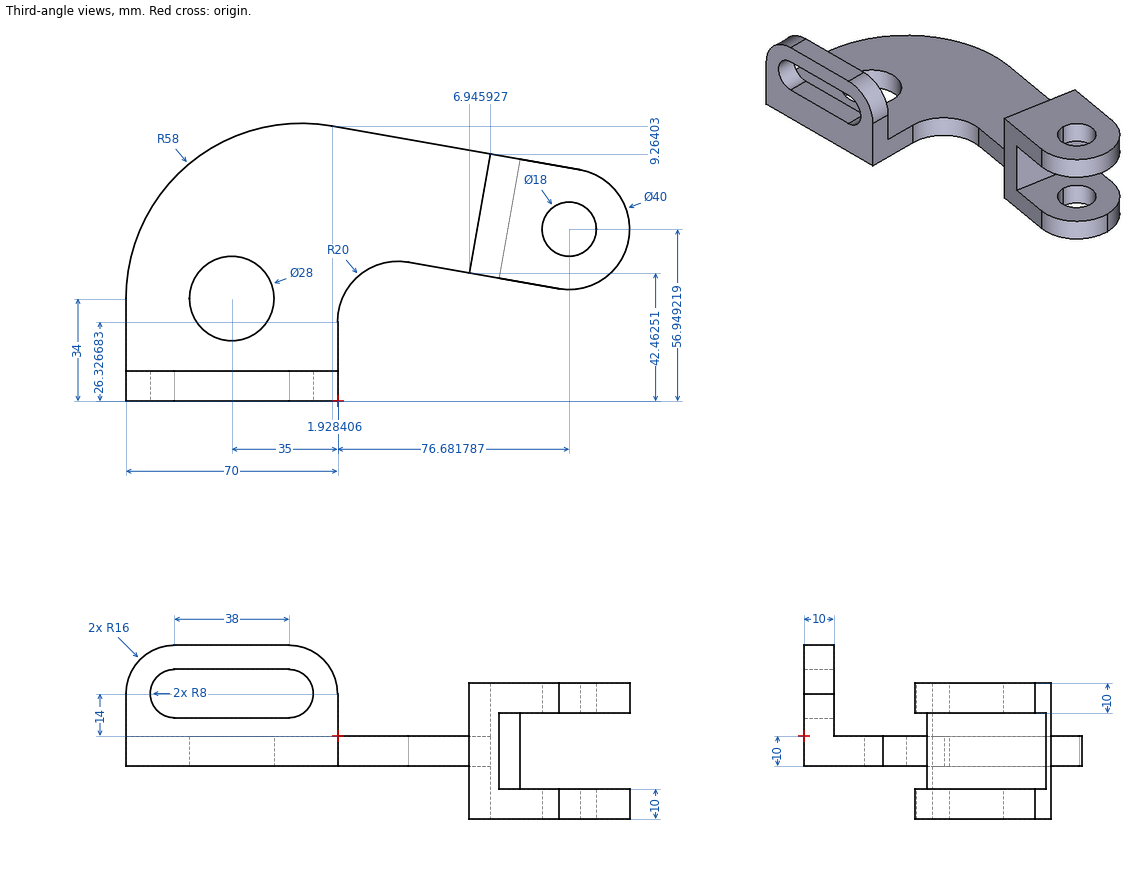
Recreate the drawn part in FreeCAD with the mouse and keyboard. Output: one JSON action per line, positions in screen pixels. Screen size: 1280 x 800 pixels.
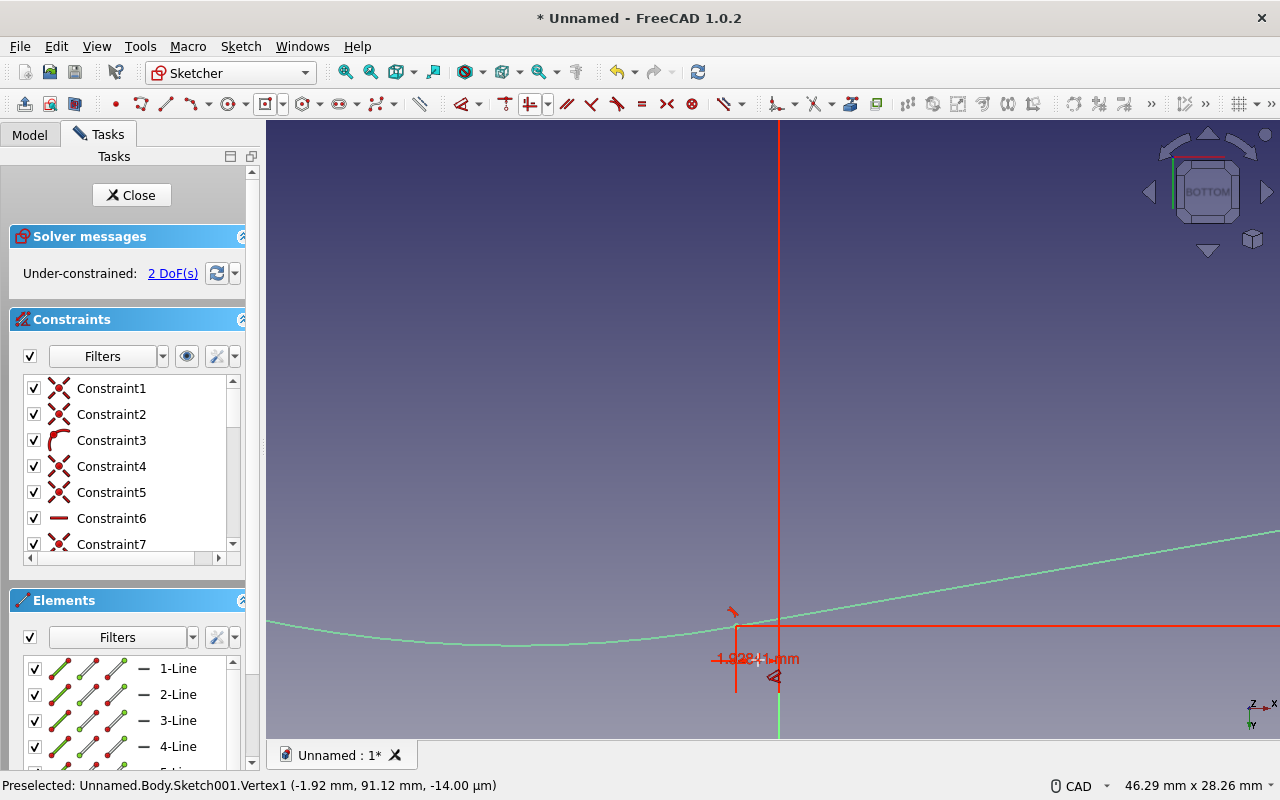
{"action": "scroll", "coordinate": [739, 632], "scroll_direction": "down", "scroll_amount": 8}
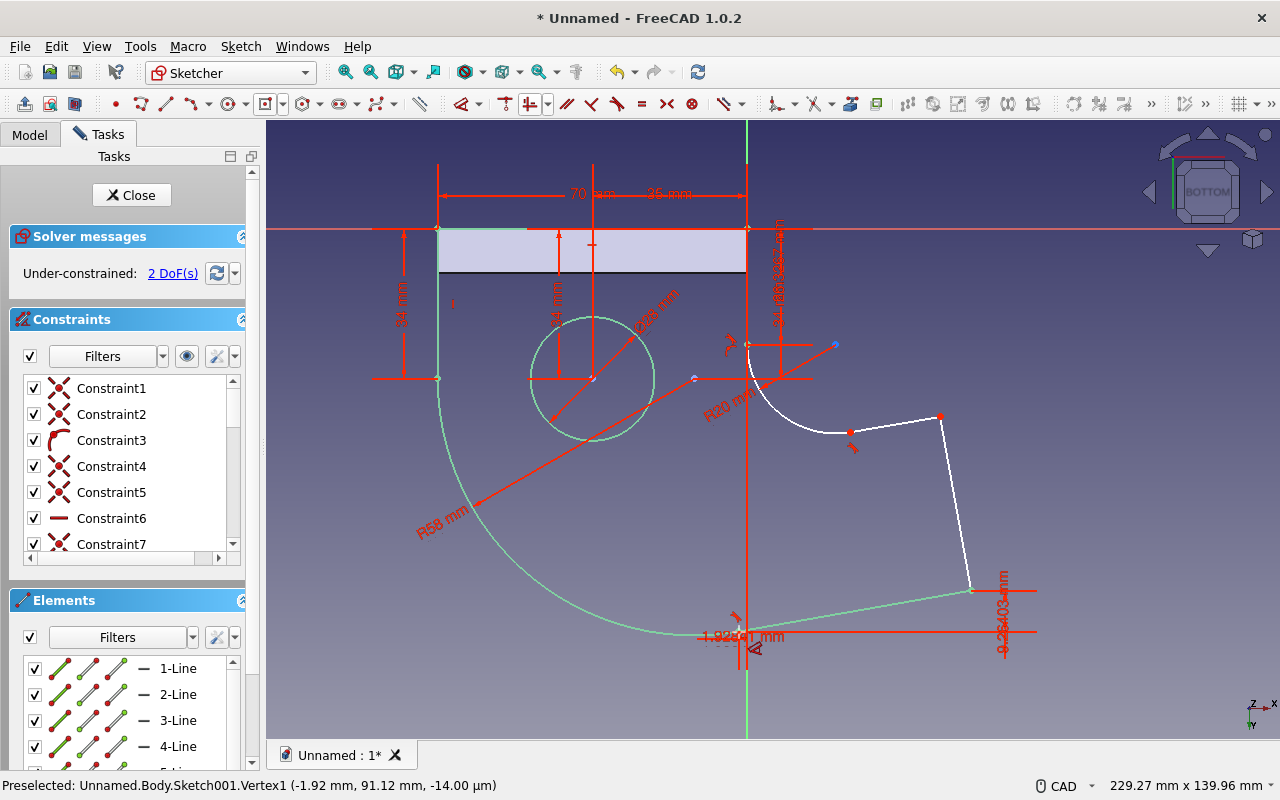
{"action": "left_click", "coordinate": [940, 417]}
{"action": "left_click", "coordinate": [974, 323]}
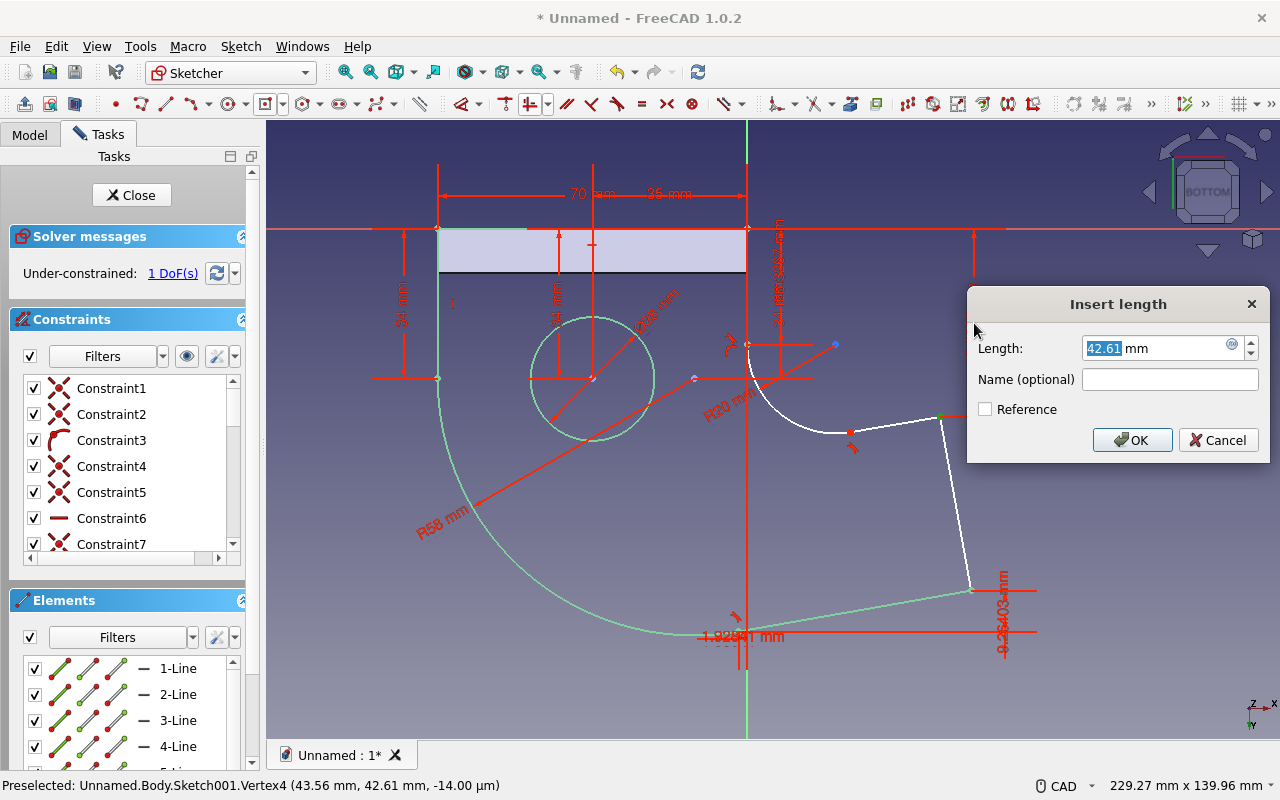
{"action": "type", "text": "42.46251"}
{"action": "key", "text": "Return"}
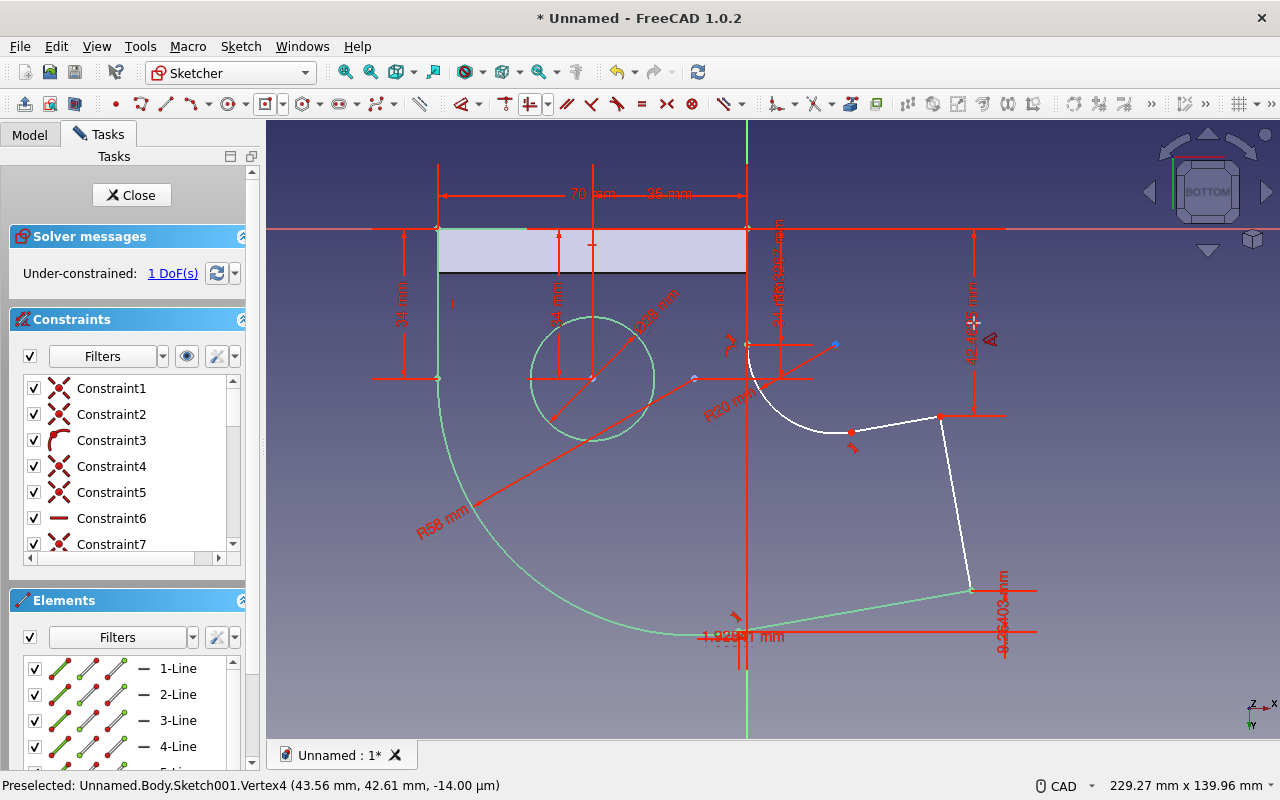
{"action": "scroll", "coordinate": [962, 538], "scroll_direction": "up", "scroll_amount": 2}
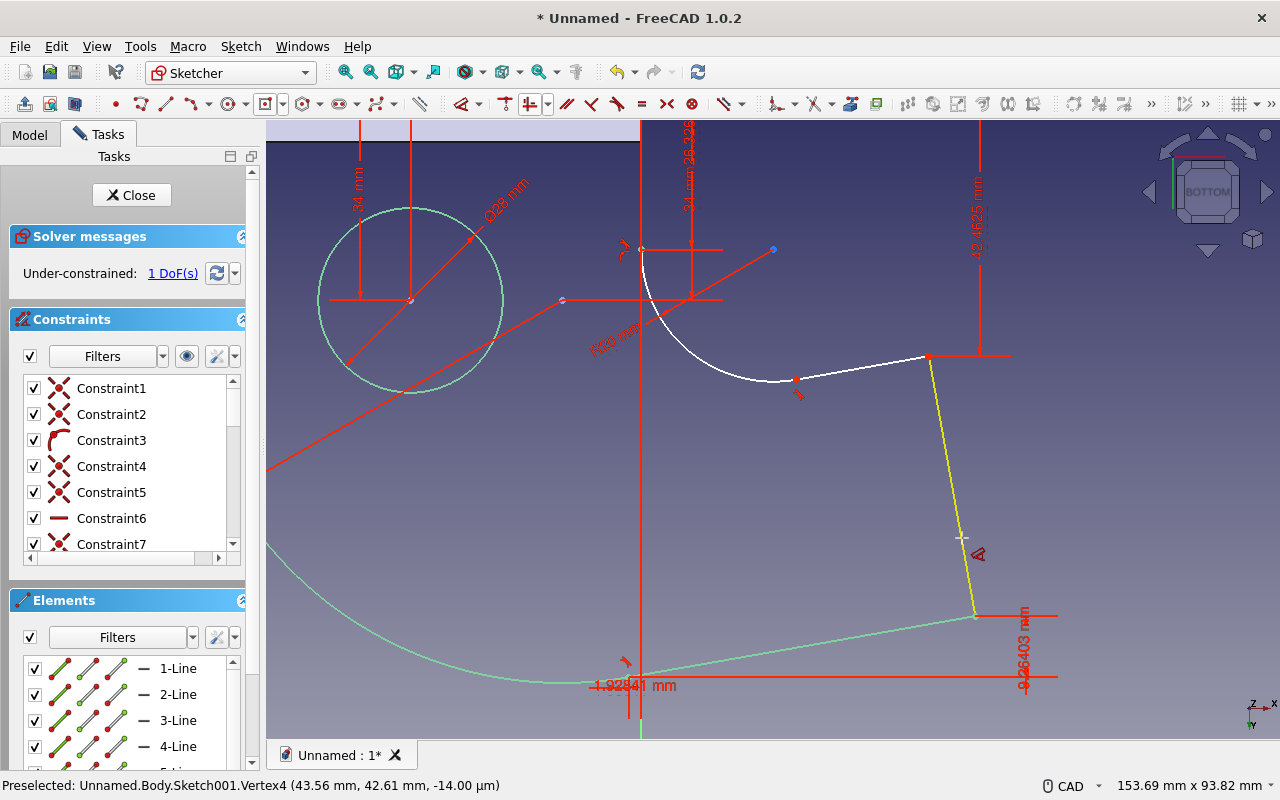
{"action": "left_click", "coordinate": [961, 538]}
{"action": "left_click", "coordinate": [952, 650]}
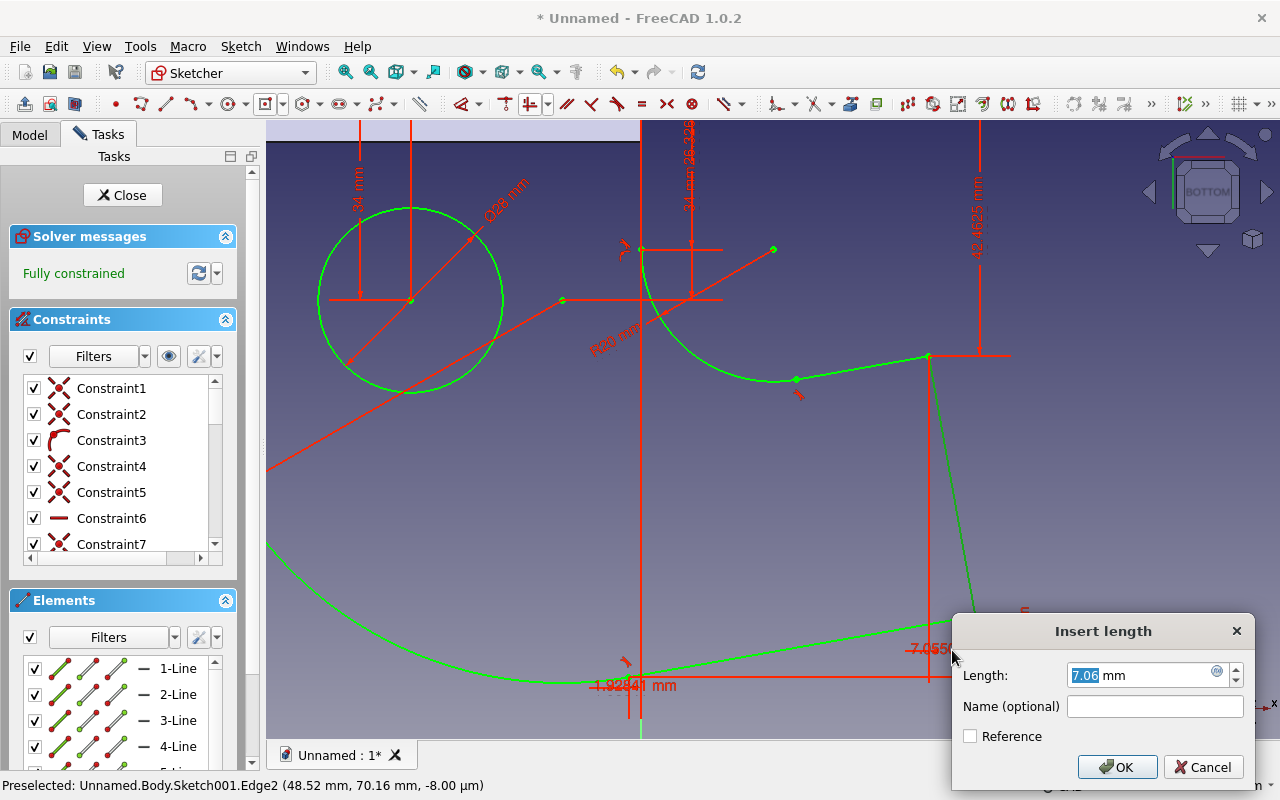
{"action": "type", "text": "6.945927"}
{"action": "key", "text": "Return"}
{"action": "key", "text": "Escape"}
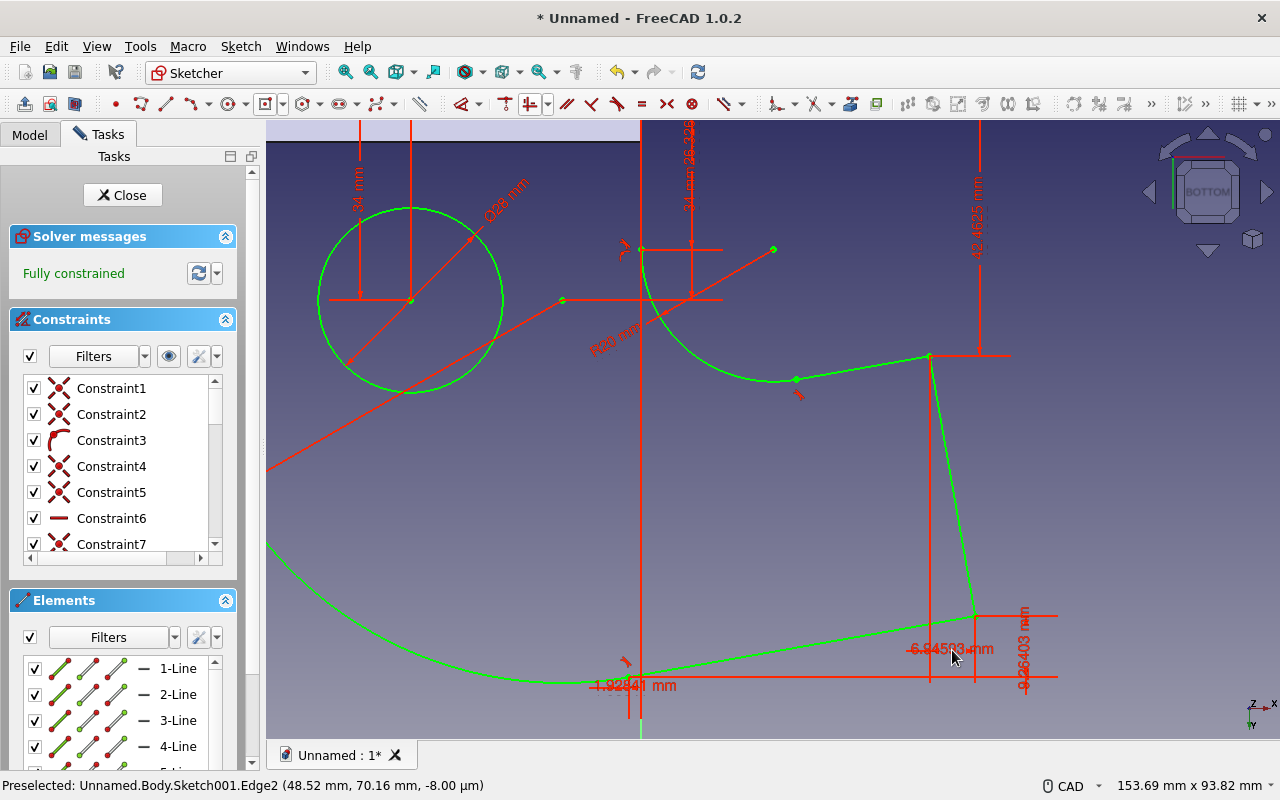
{"action": "left_click", "coordinate": [123, 195]}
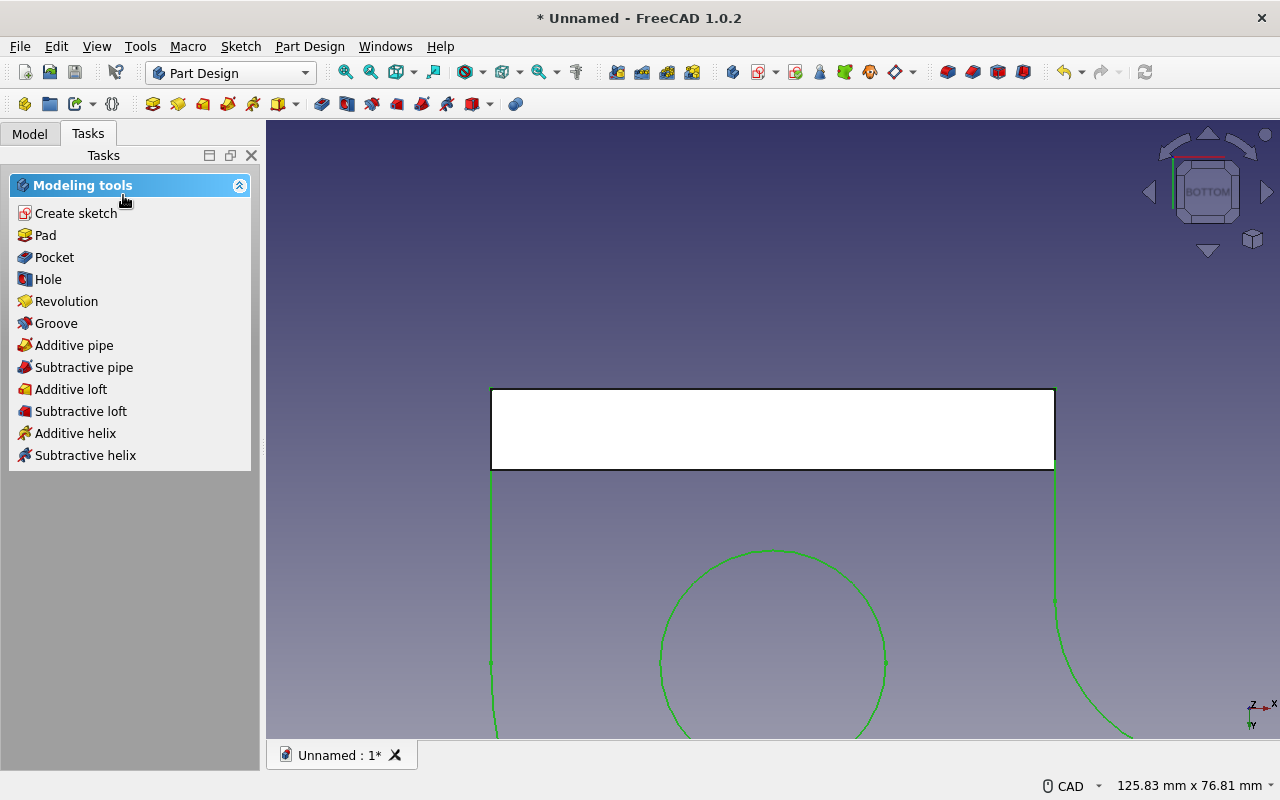
{"action": "left_click", "coordinate": [153, 104]}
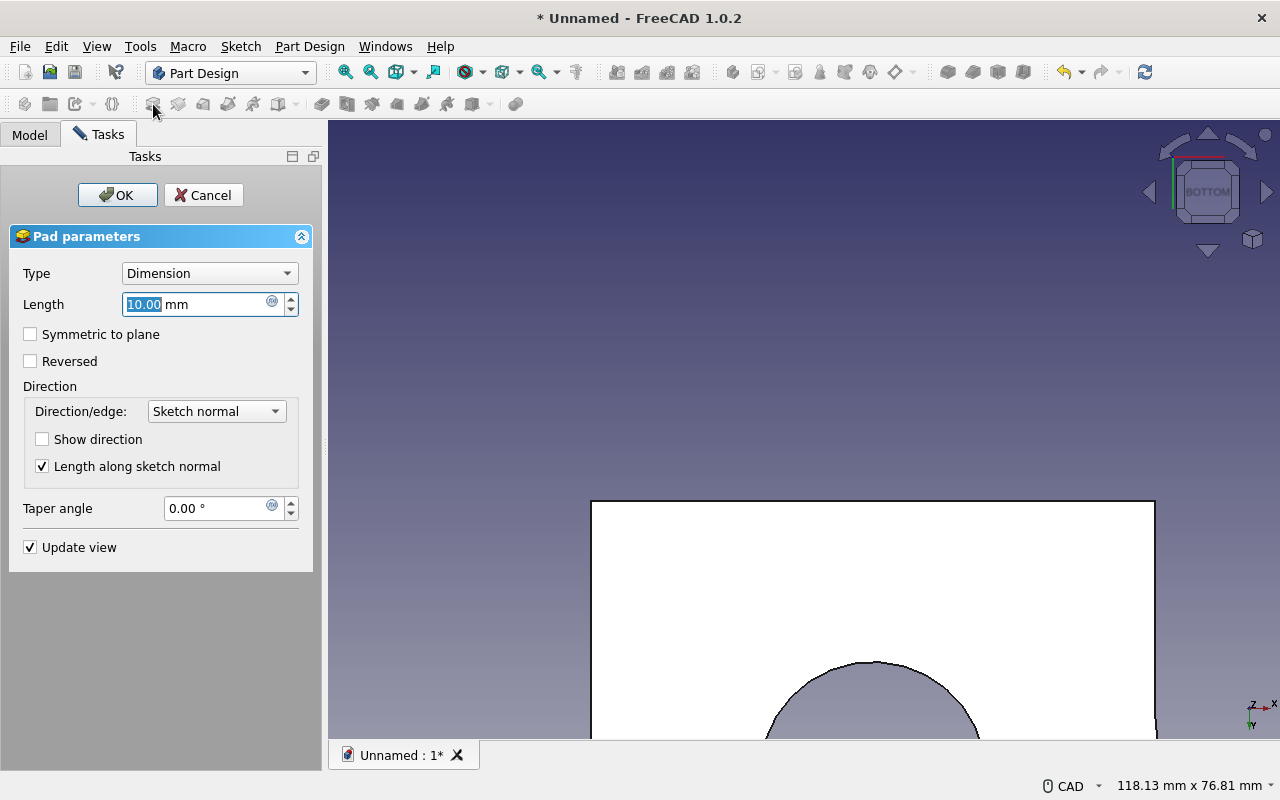
{"action": "type", "text": "10"}
{"action": "key", "text": "Tab"}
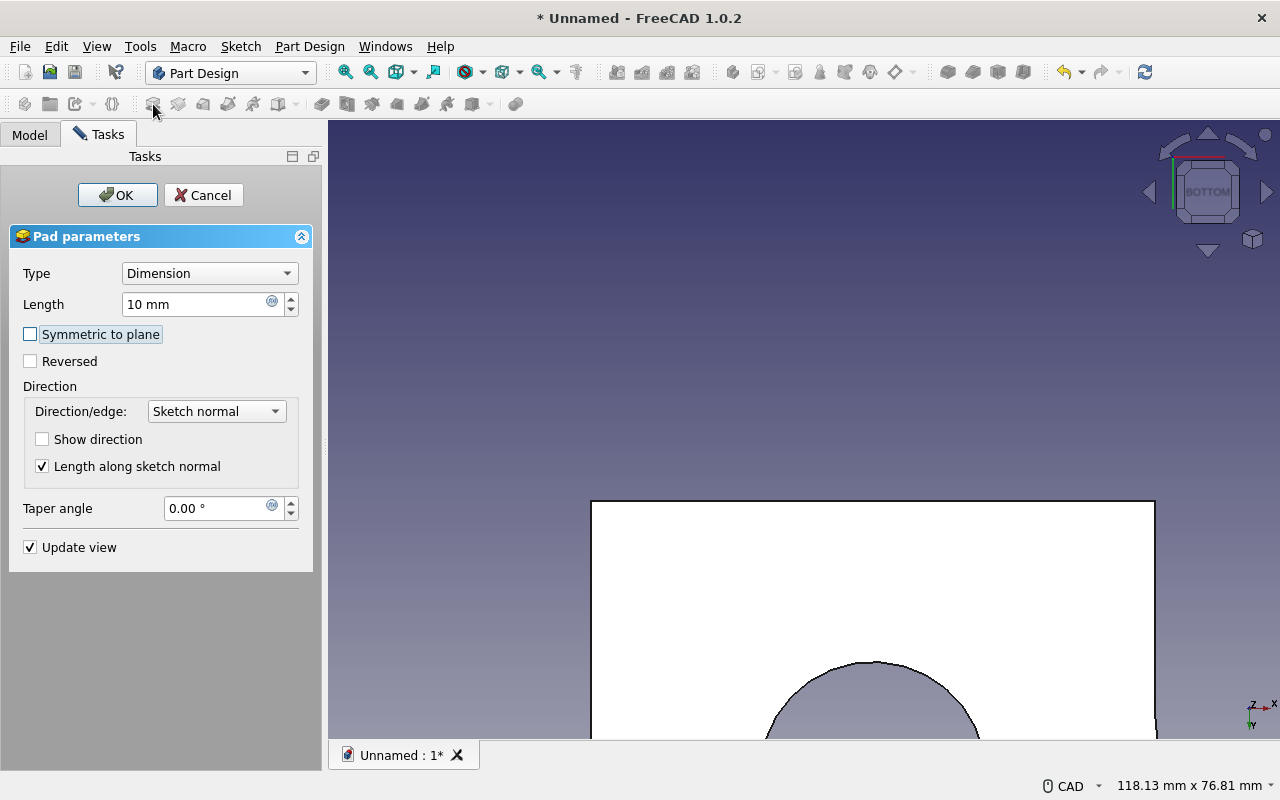
{"action": "left_click", "coordinate": [118, 195]}